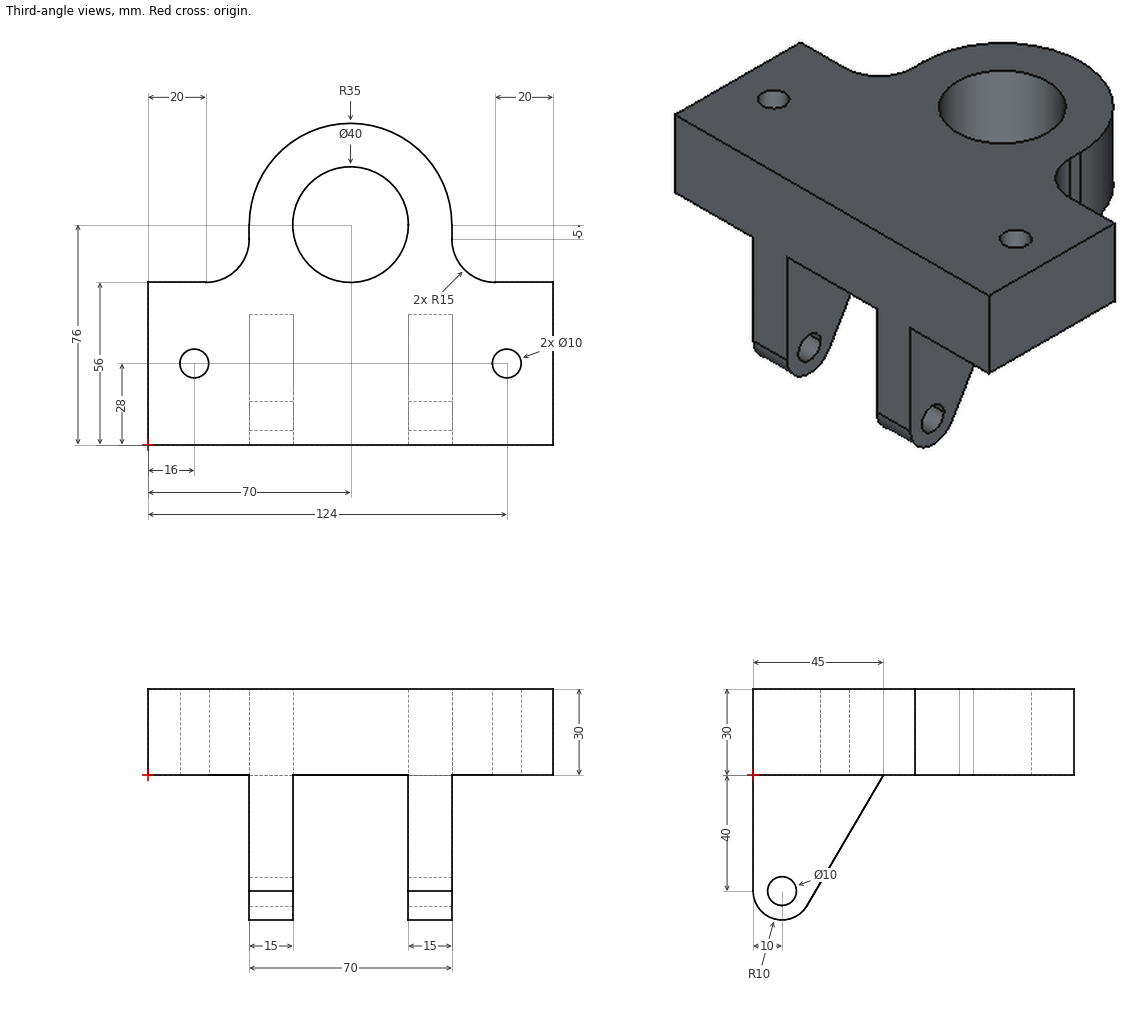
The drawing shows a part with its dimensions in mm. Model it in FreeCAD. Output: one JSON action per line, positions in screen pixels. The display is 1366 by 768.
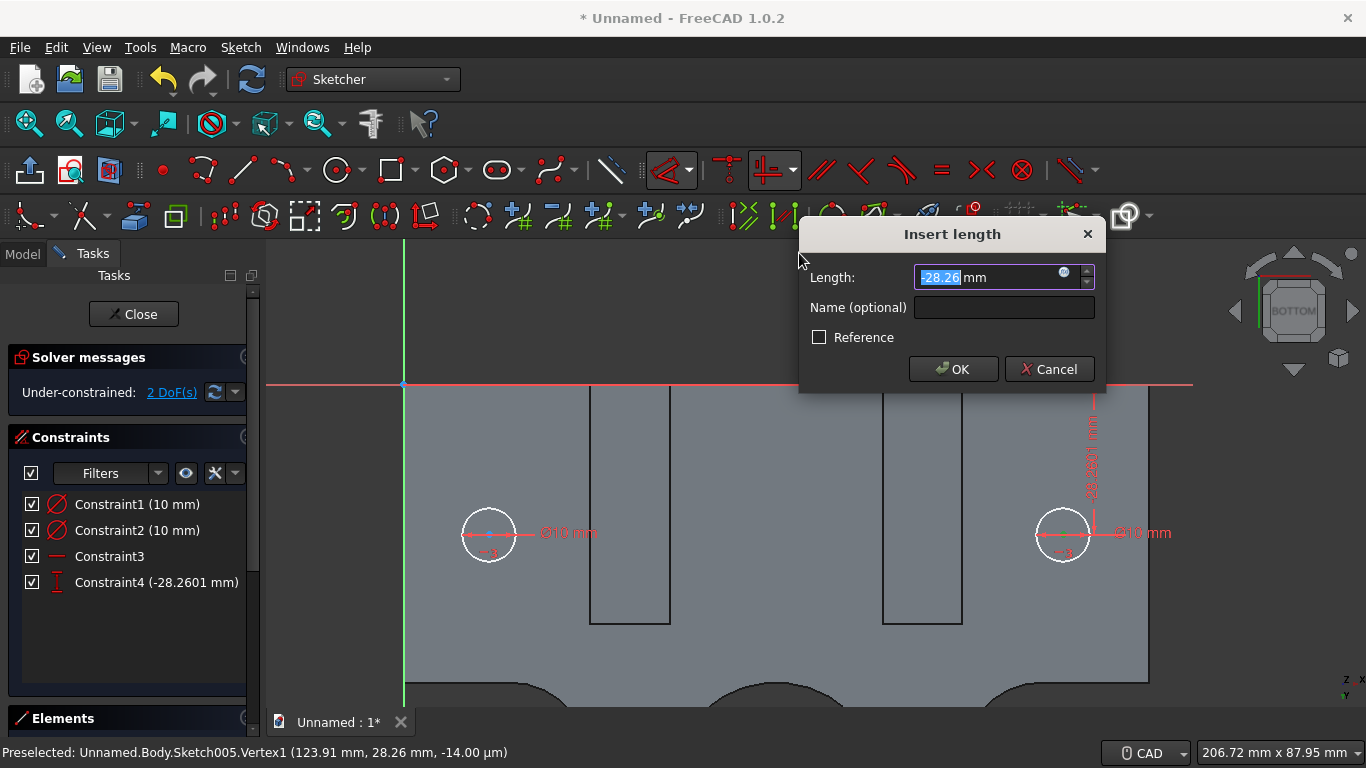
{"action": "type", "text": "-28"}
{"action": "key", "text": "Return"}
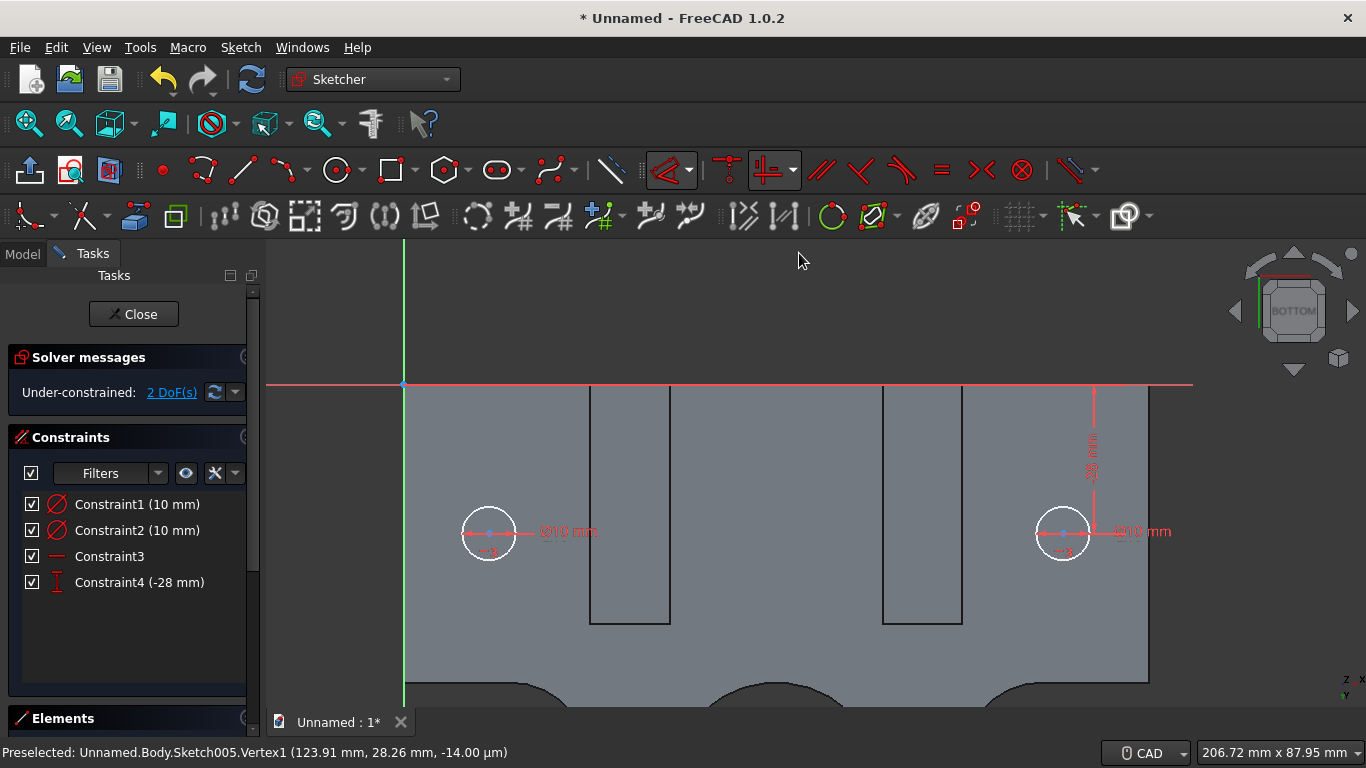
{"action": "left_click", "coordinate": [489, 534]}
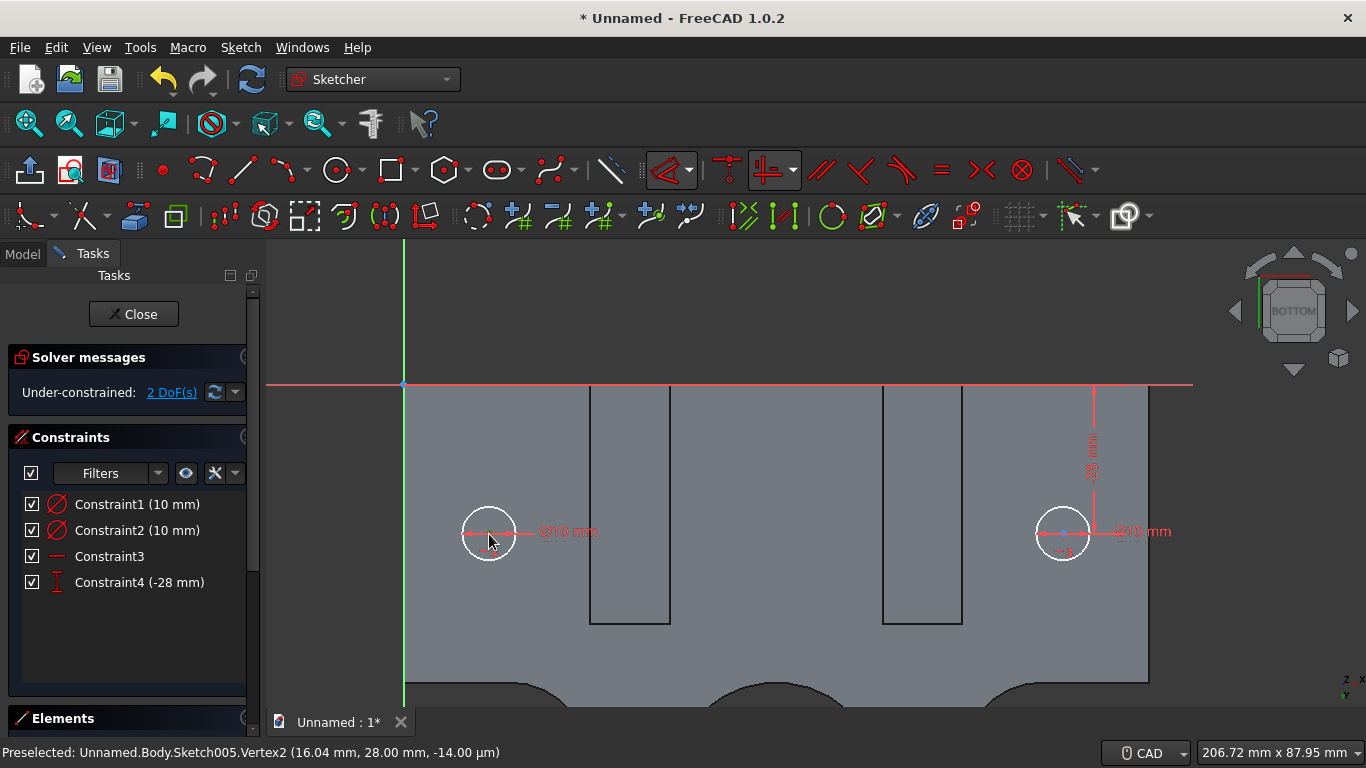
{"action": "left_click", "coordinate": [692, 170]}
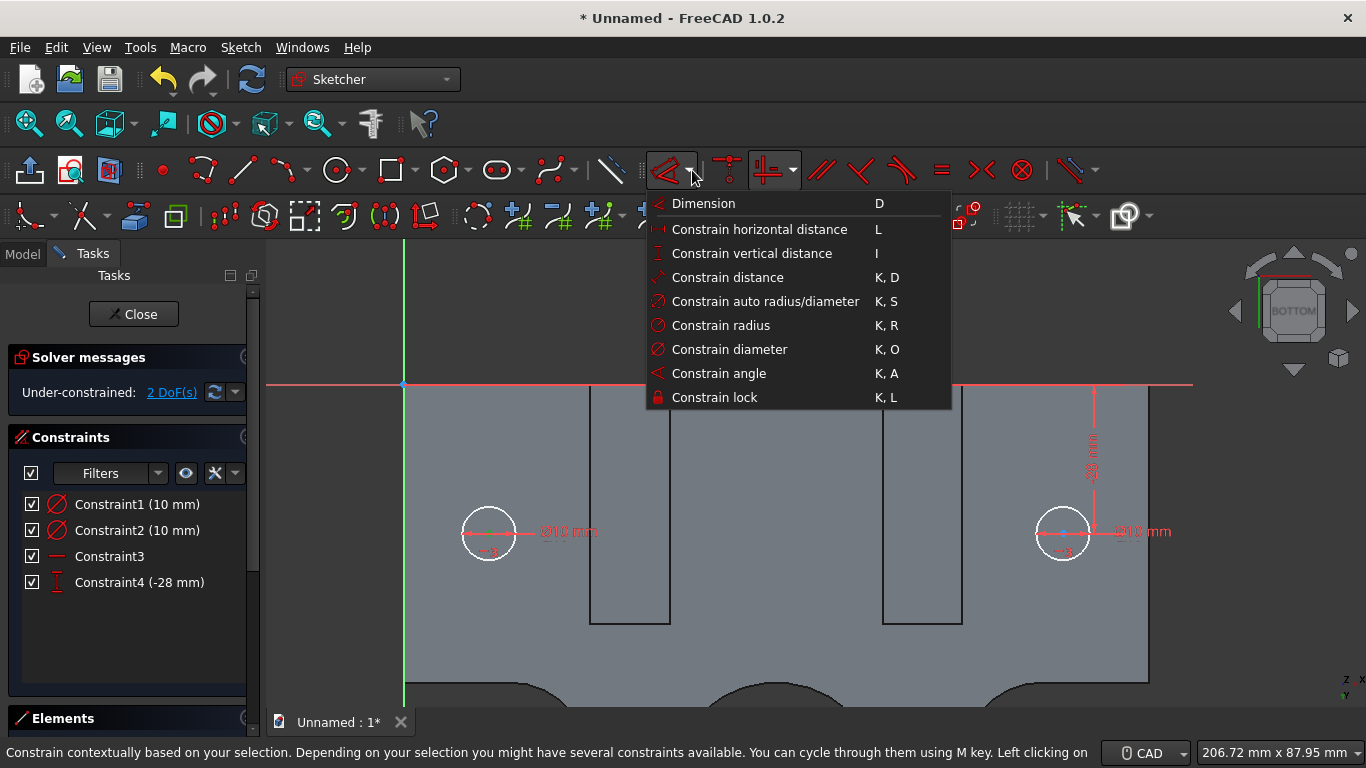
{"action": "left_click", "coordinate": [799, 229]}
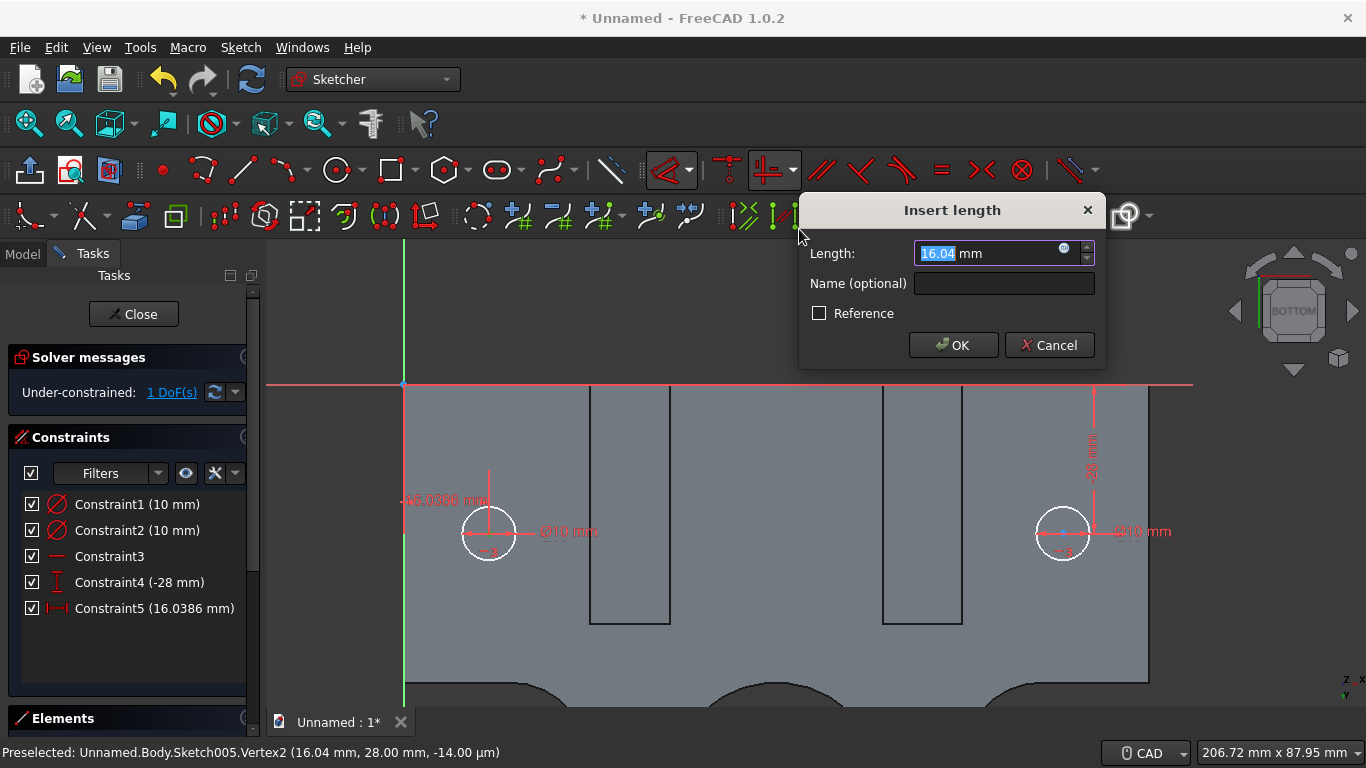
{"action": "type", "text": "16"}
{"action": "key", "text": "Return"}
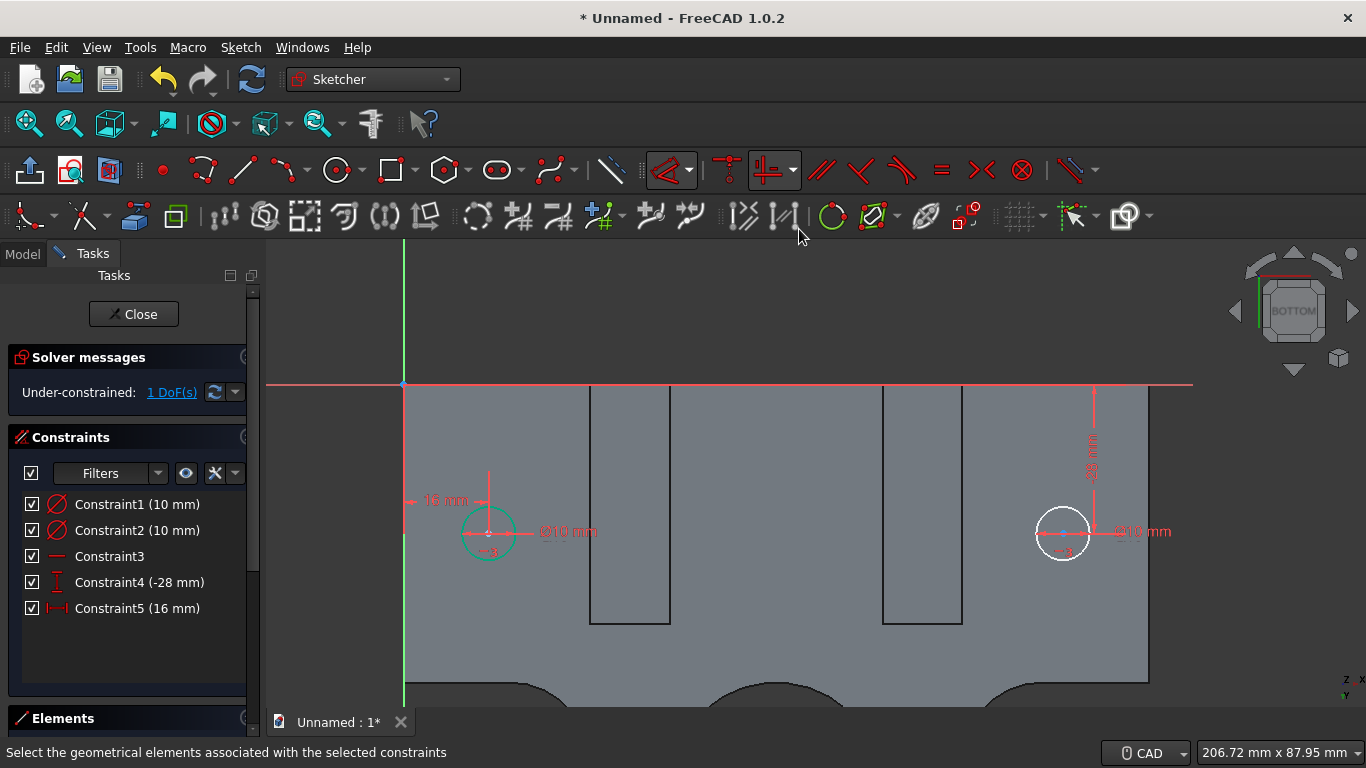
{"action": "left_click", "coordinate": [1063, 534]}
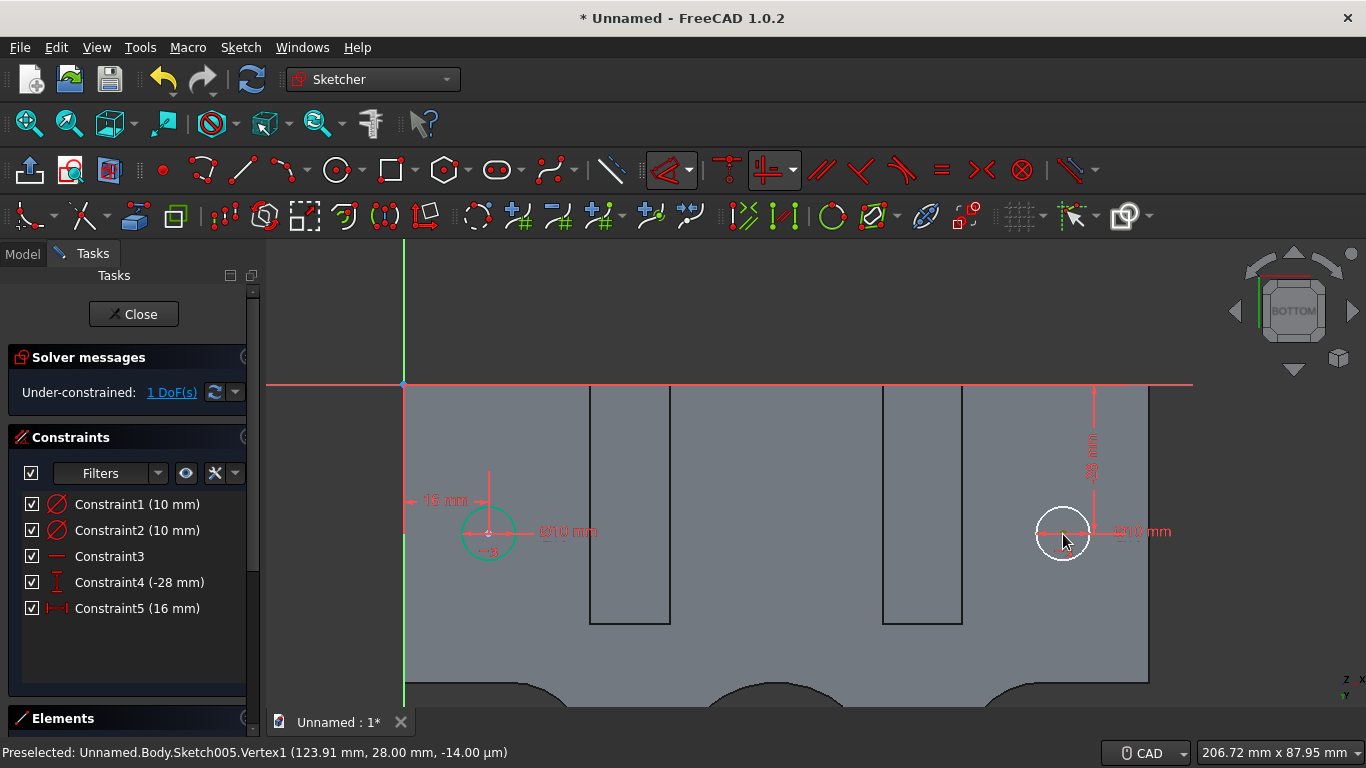
{"action": "left_click", "coordinate": [692, 170]}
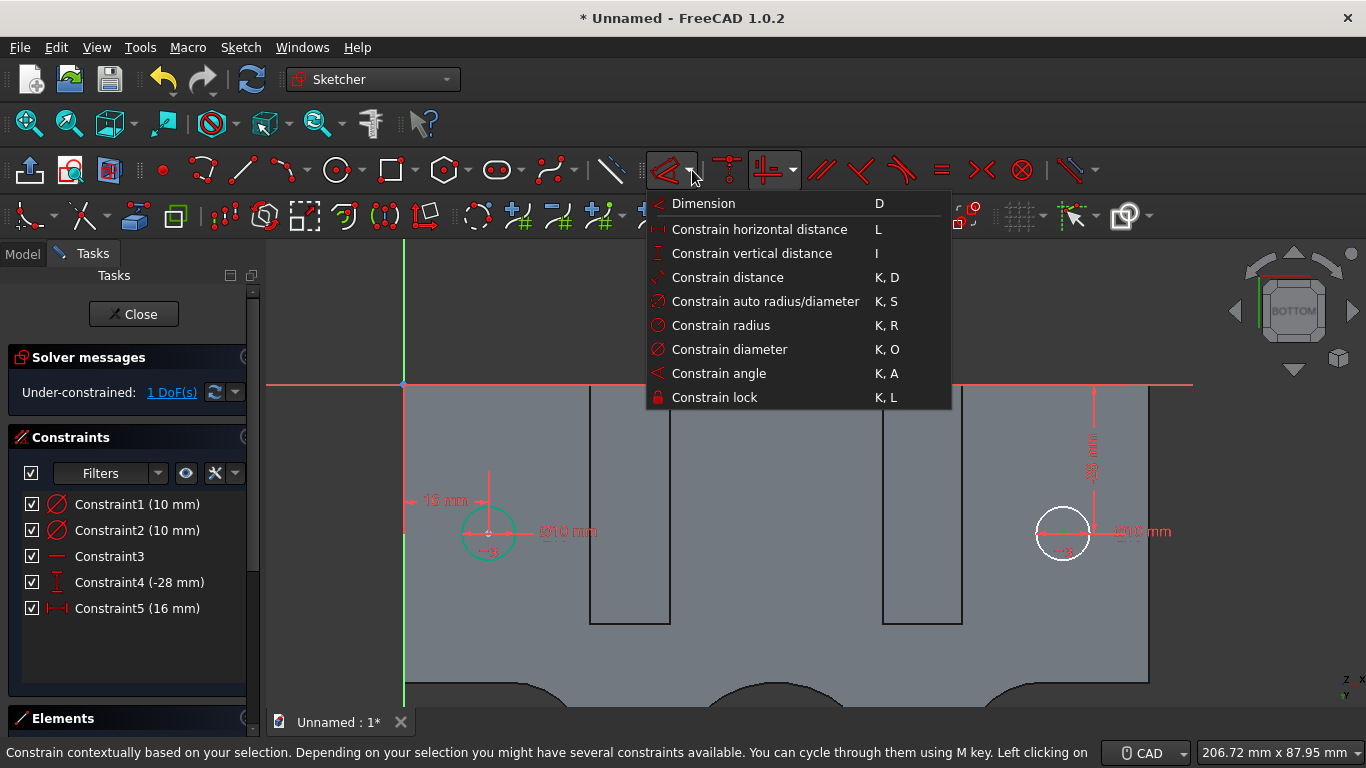
{"action": "left_click", "coordinate": [799, 229]}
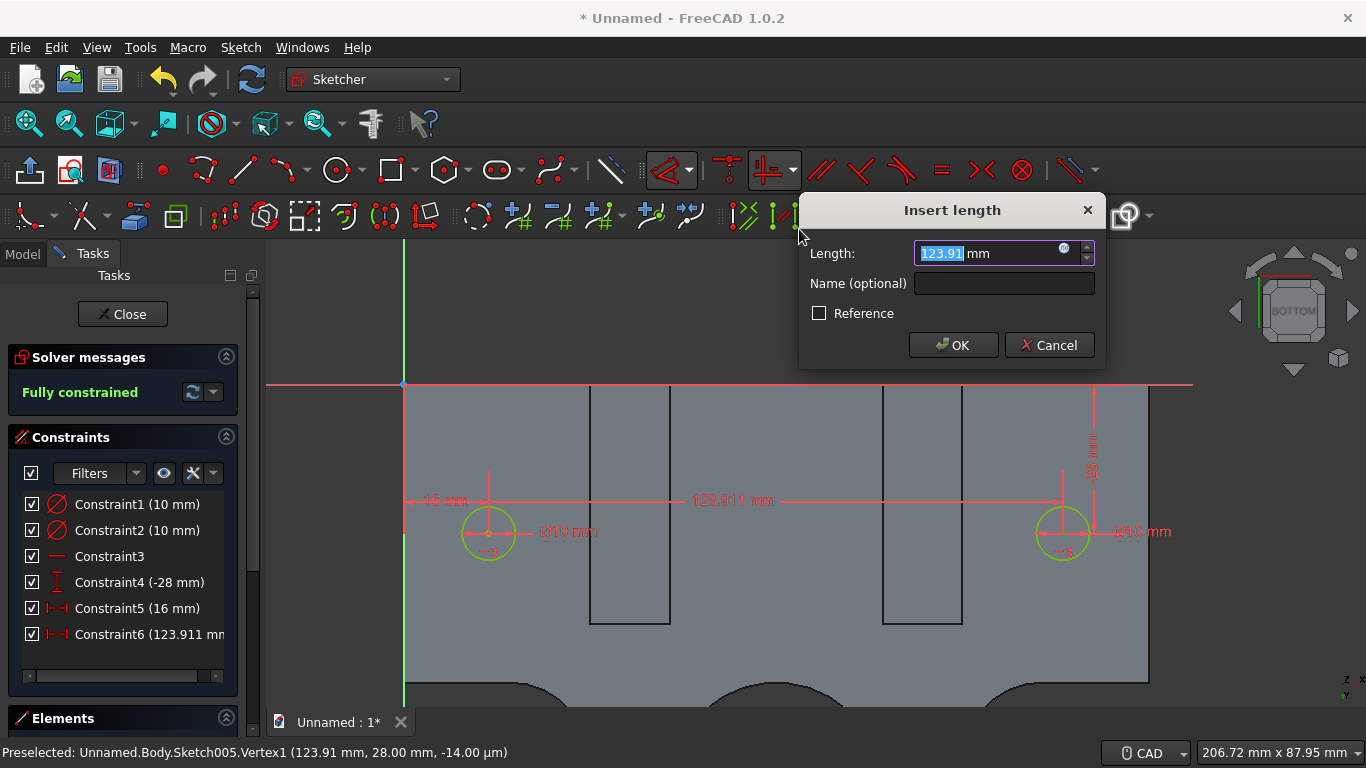
{"action": "type", "text": "124"}
{"action": "key", "text": "Return"}